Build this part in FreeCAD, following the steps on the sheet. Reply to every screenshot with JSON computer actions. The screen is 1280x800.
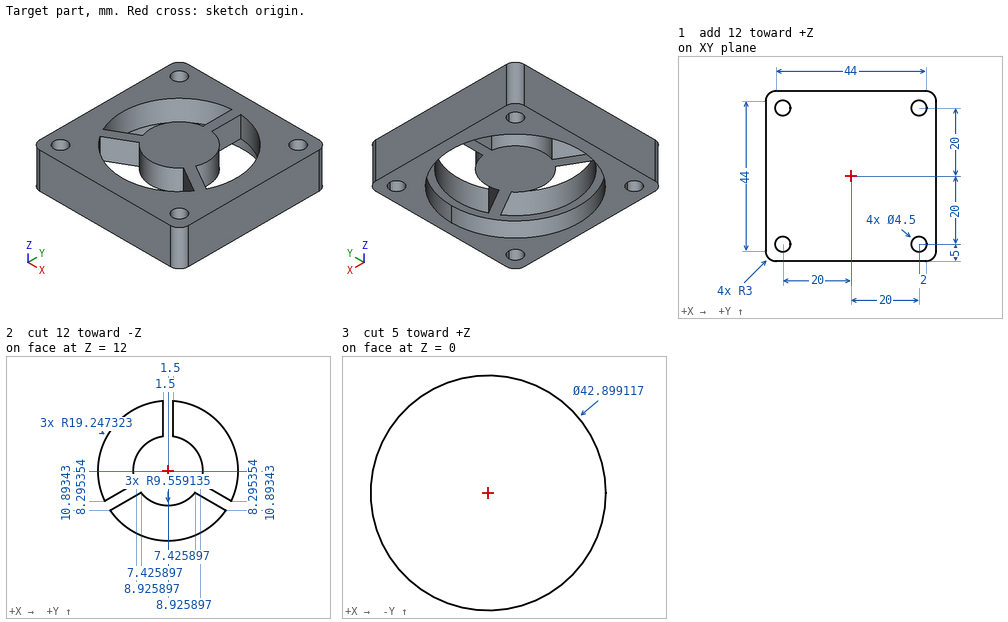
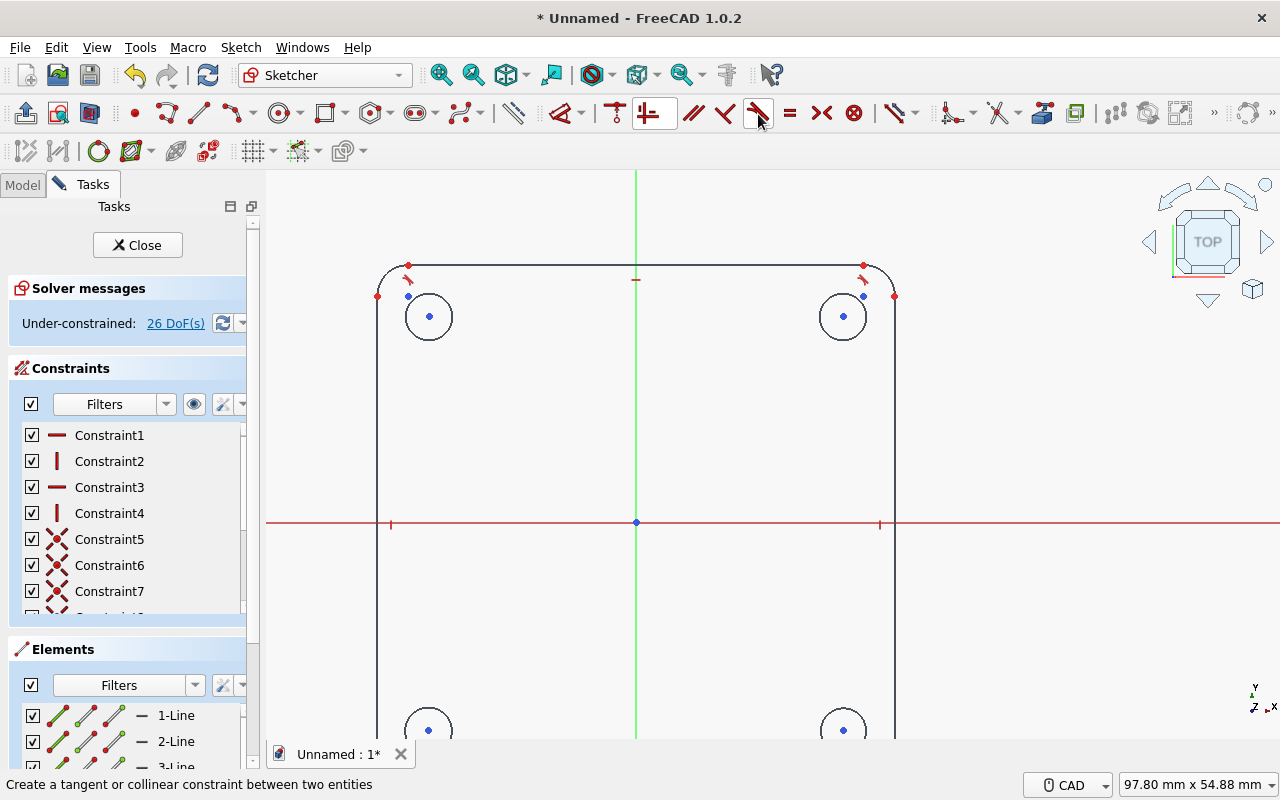
{"action": "left_click", "coordinate": [377, 433]}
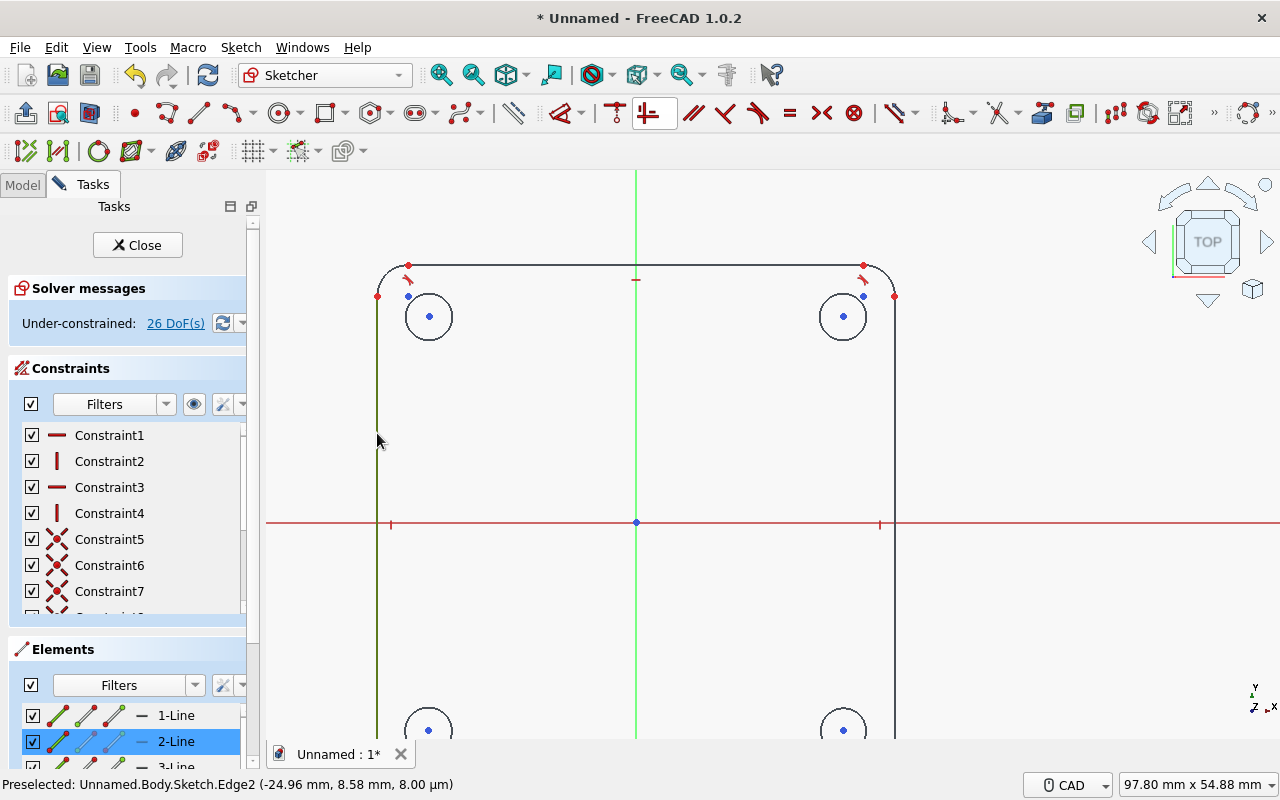
{"action": "left_click", "coordinate": [394, 269]}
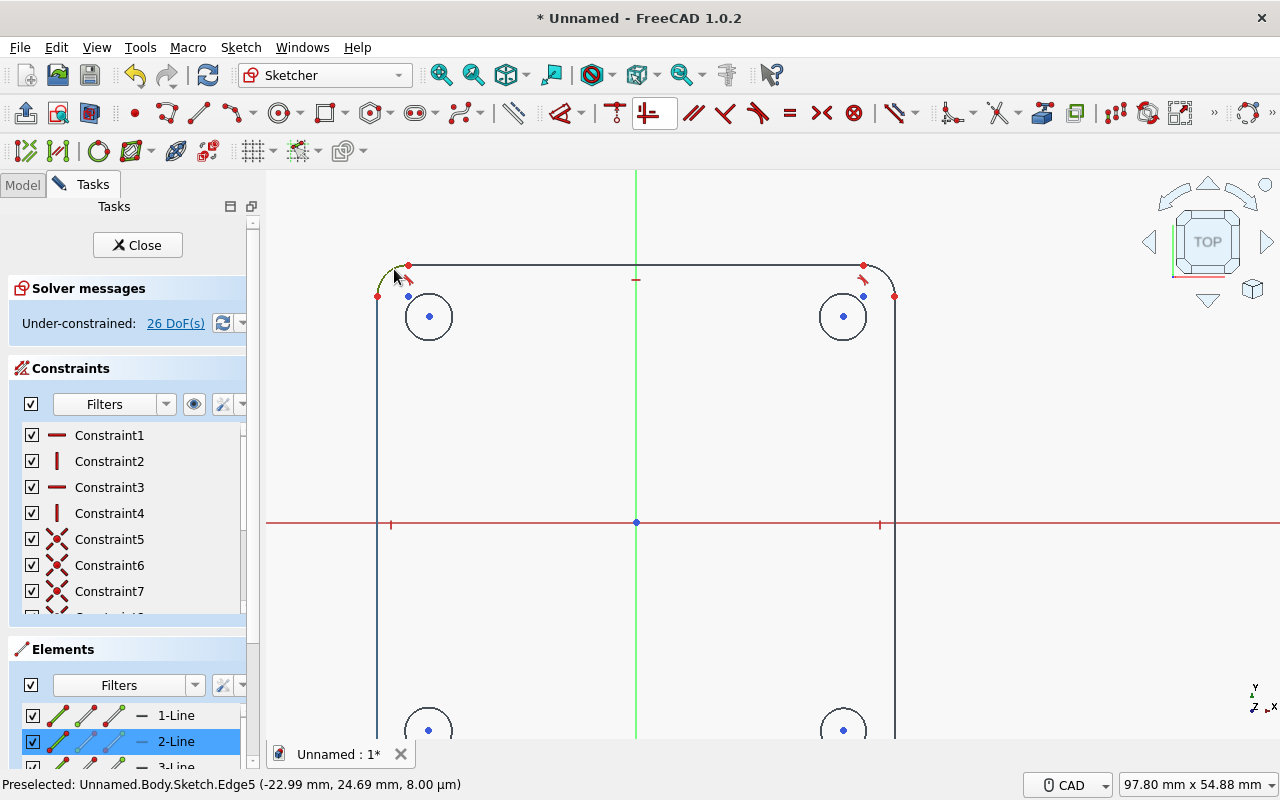
{"action": "left_click", "coordinate": [758, 114]}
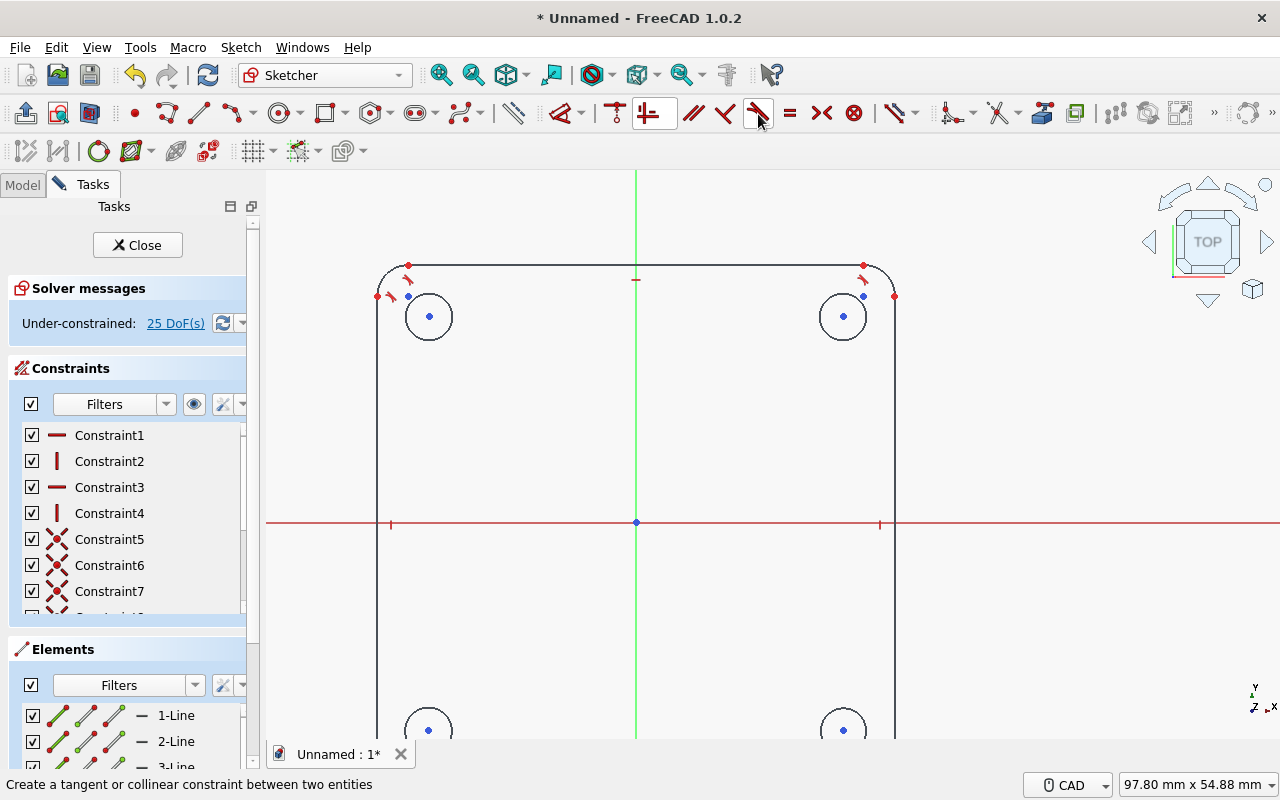
{"action": "left_click", "coordinate": [377, 433]}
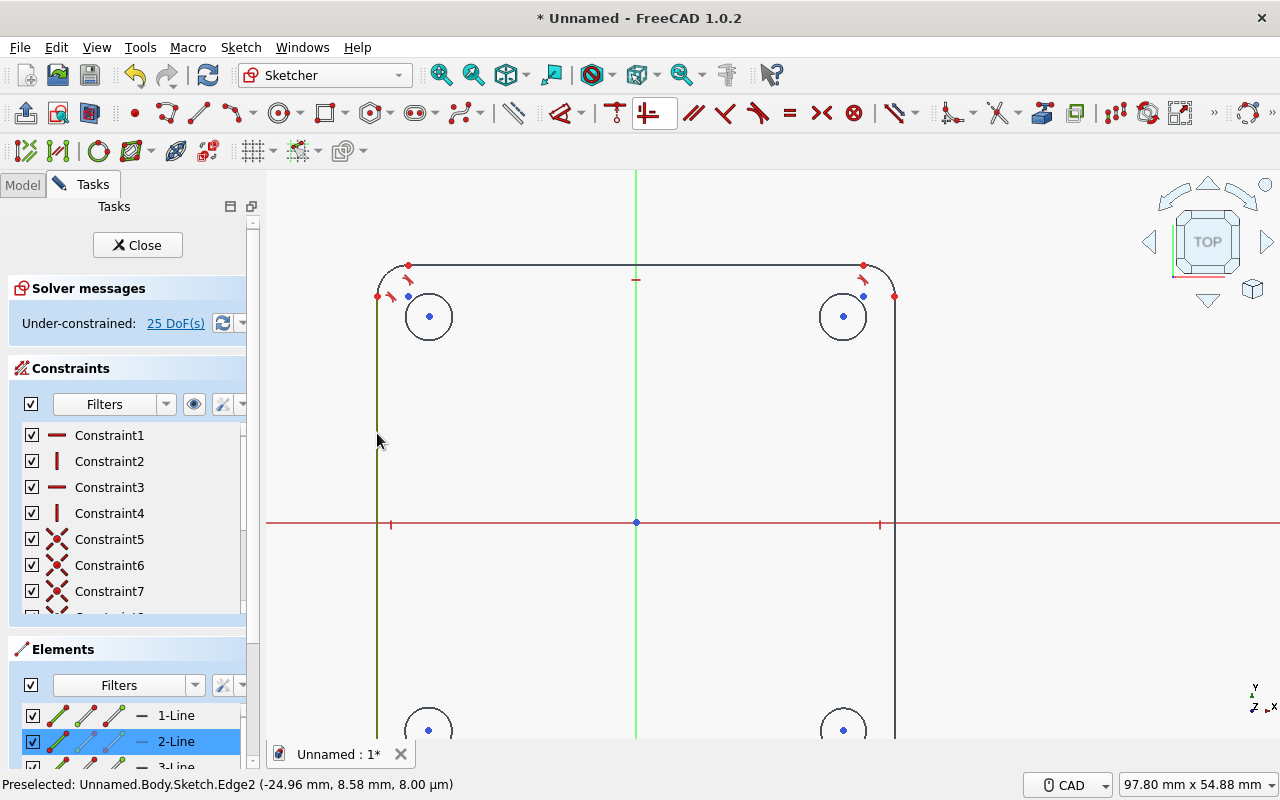
{"action": "scroll", "coordinate": [844, 315], "scroll_direction": "down", "scroll_amount": 2}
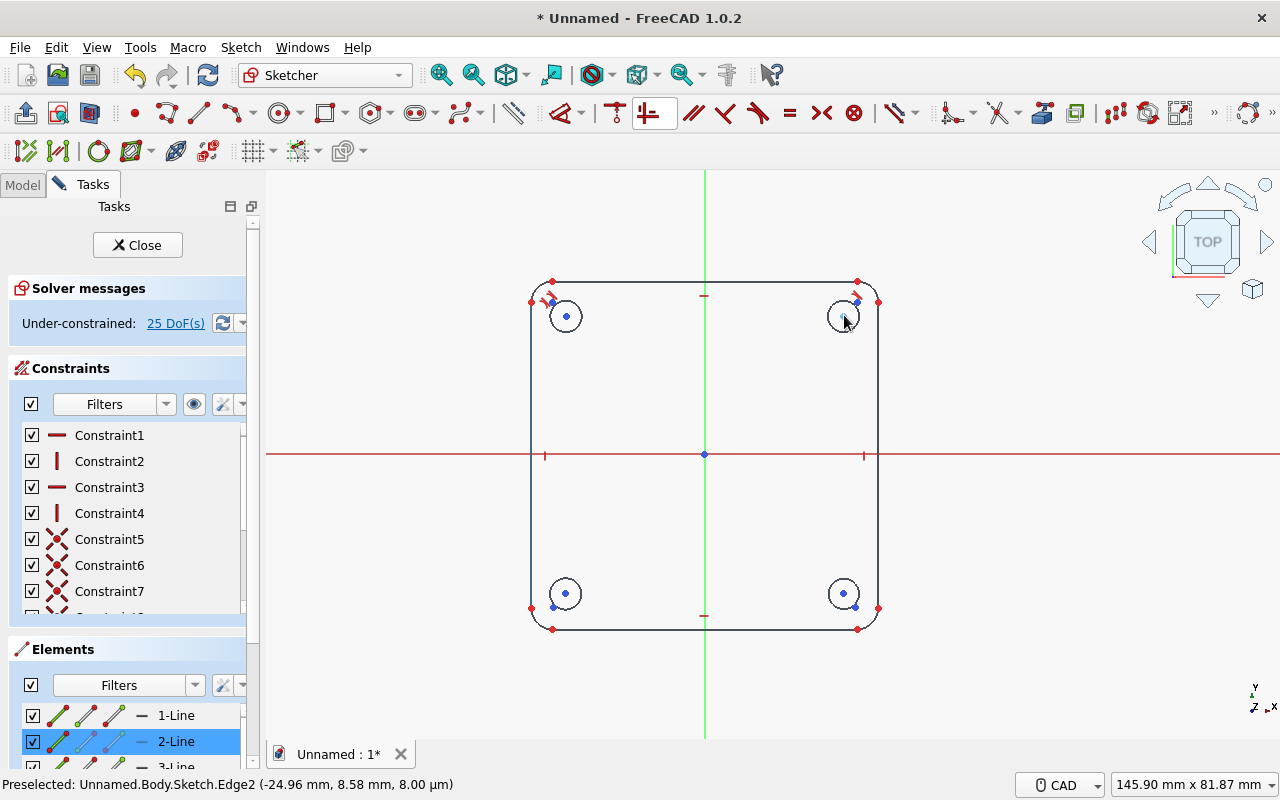
{"action": "scroll", "coordinate": [534, 618], "scroll_direction": "up", "scroll_amount": 2}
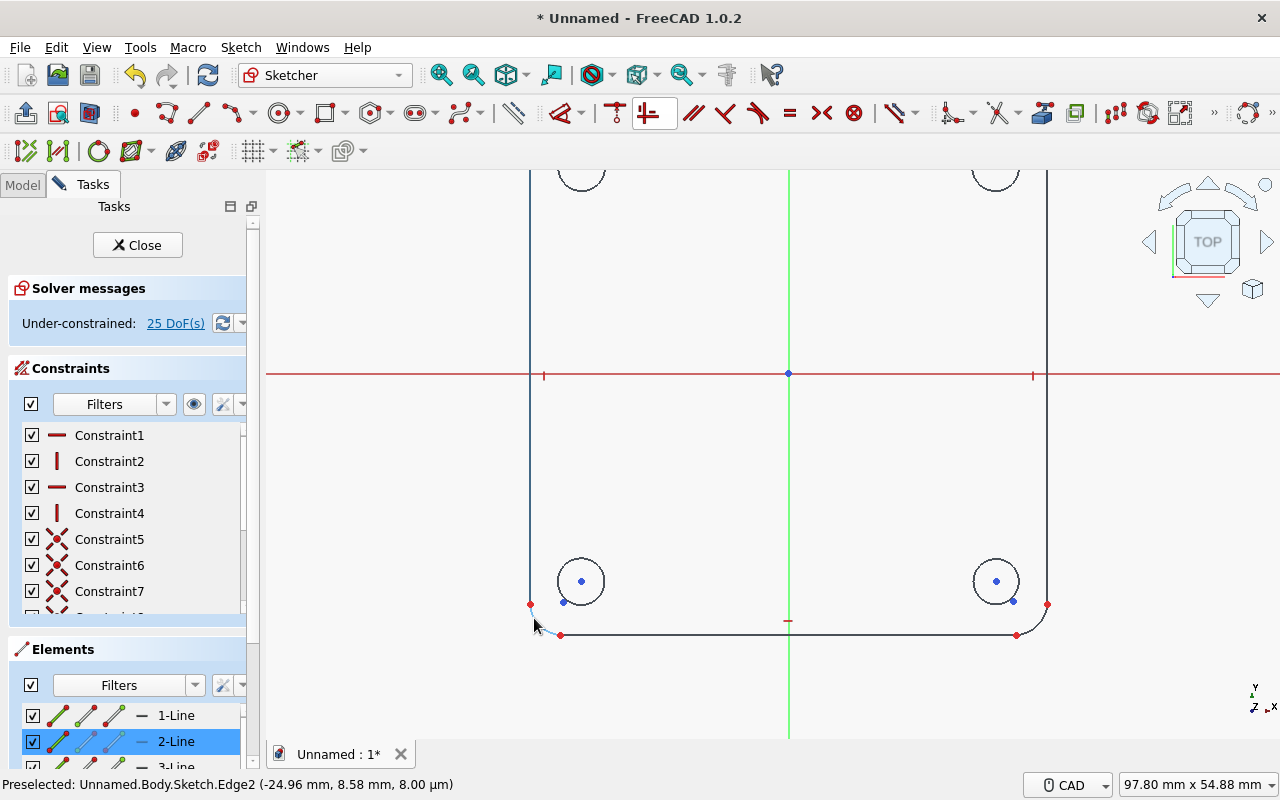
{"action": "left_click", "coordinate": [534, 618]}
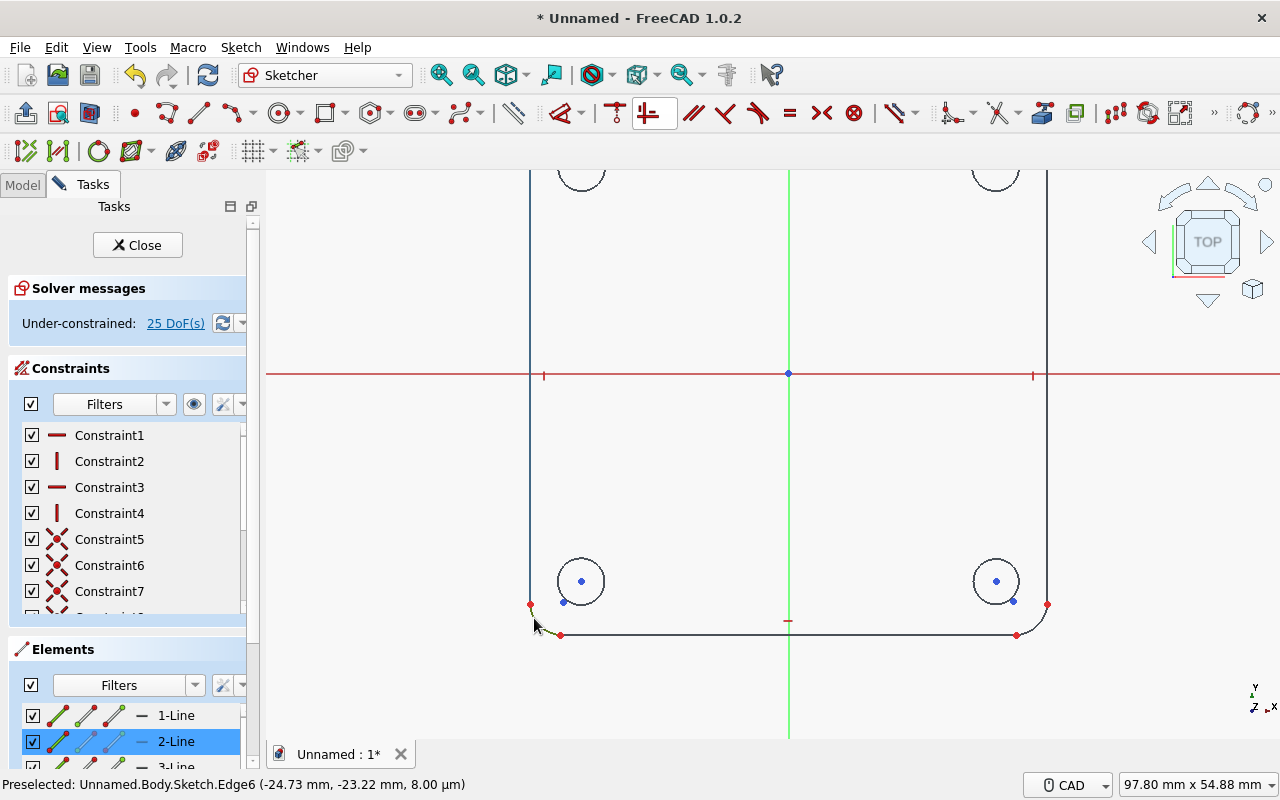
{"action": "left_click", "coordinate": [758, 114]}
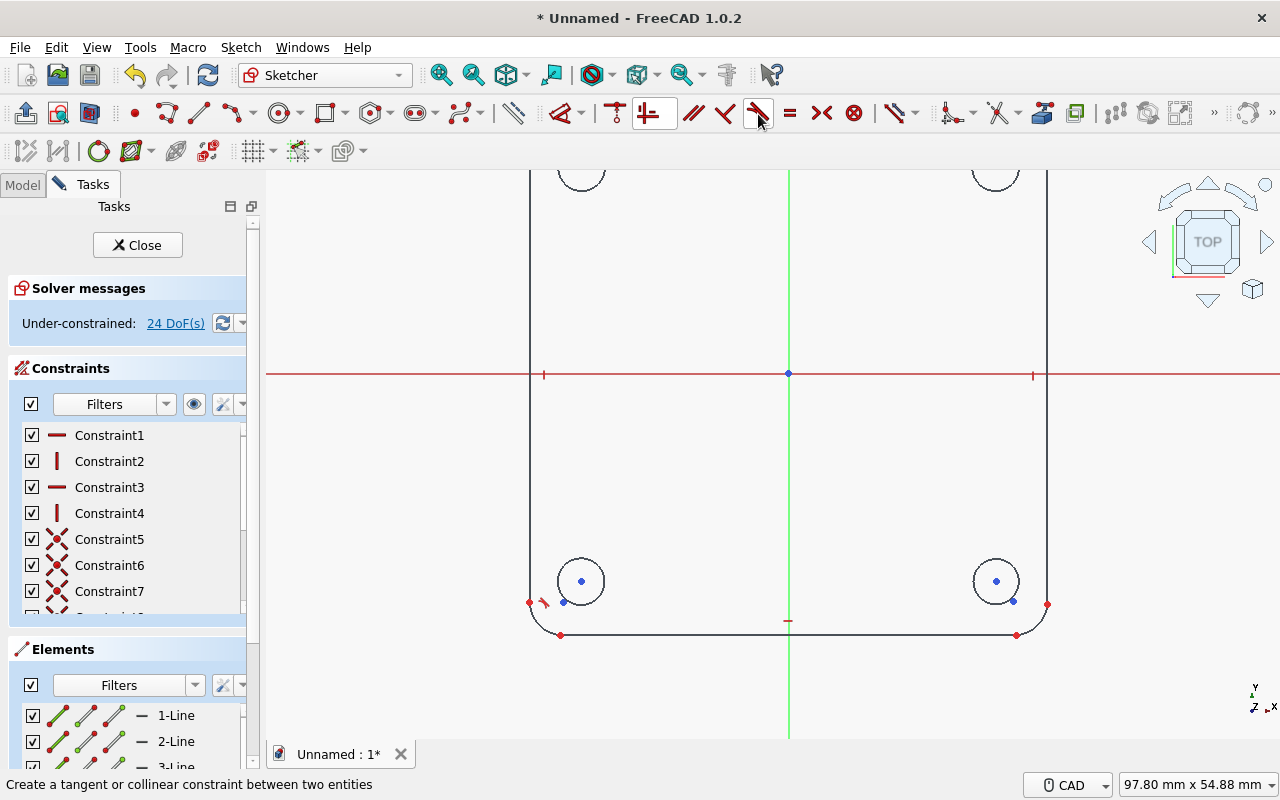
{"action": "left_click", "coordinate": [698, 635]}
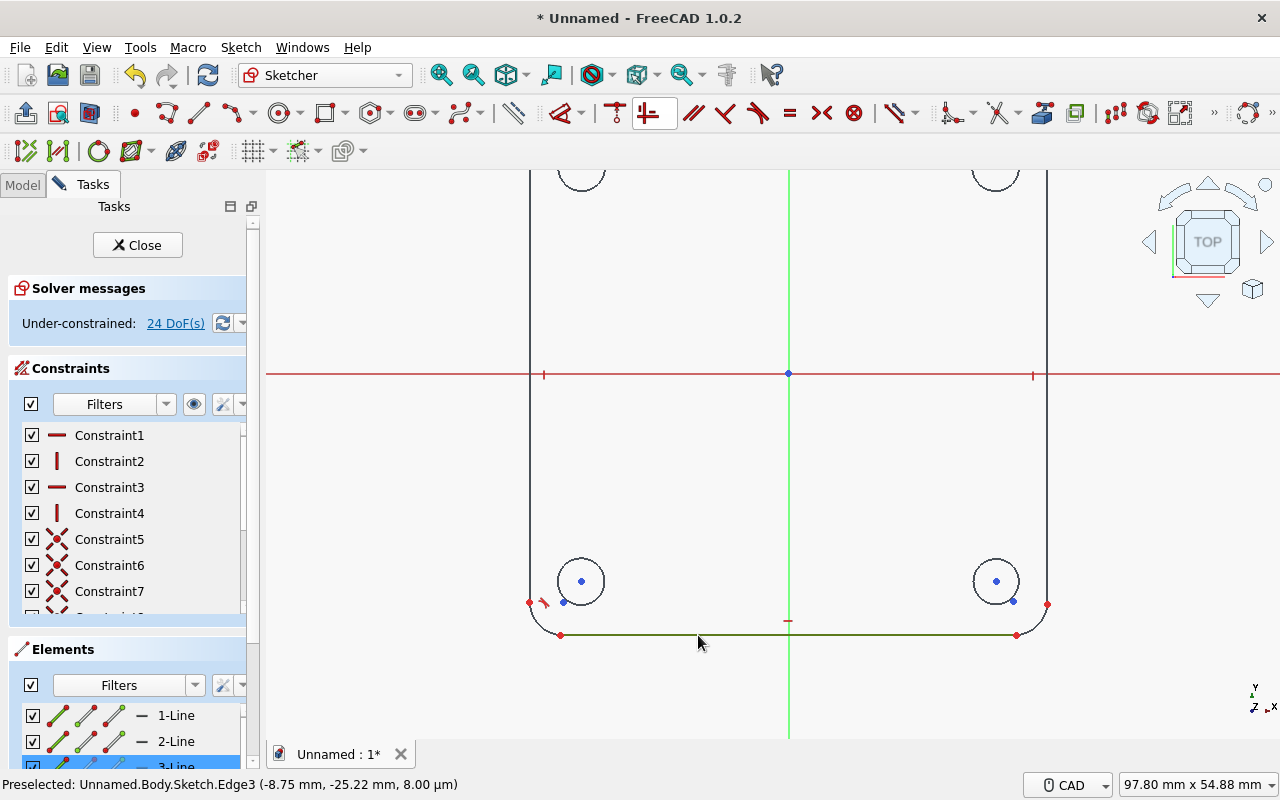
{"action": "left_click", "coordinate": [533, 617]}